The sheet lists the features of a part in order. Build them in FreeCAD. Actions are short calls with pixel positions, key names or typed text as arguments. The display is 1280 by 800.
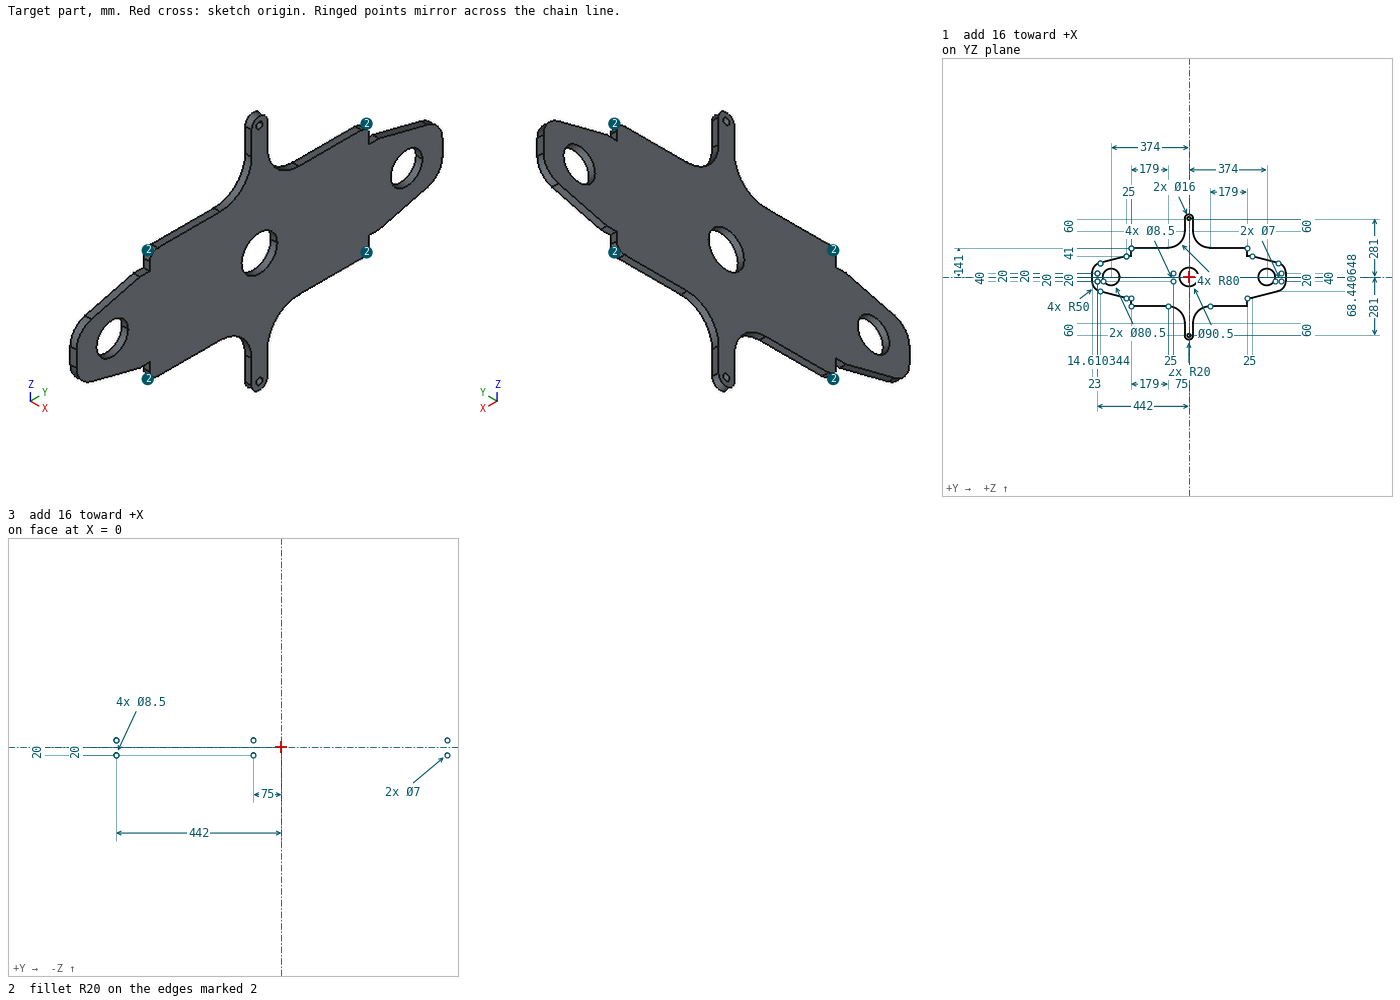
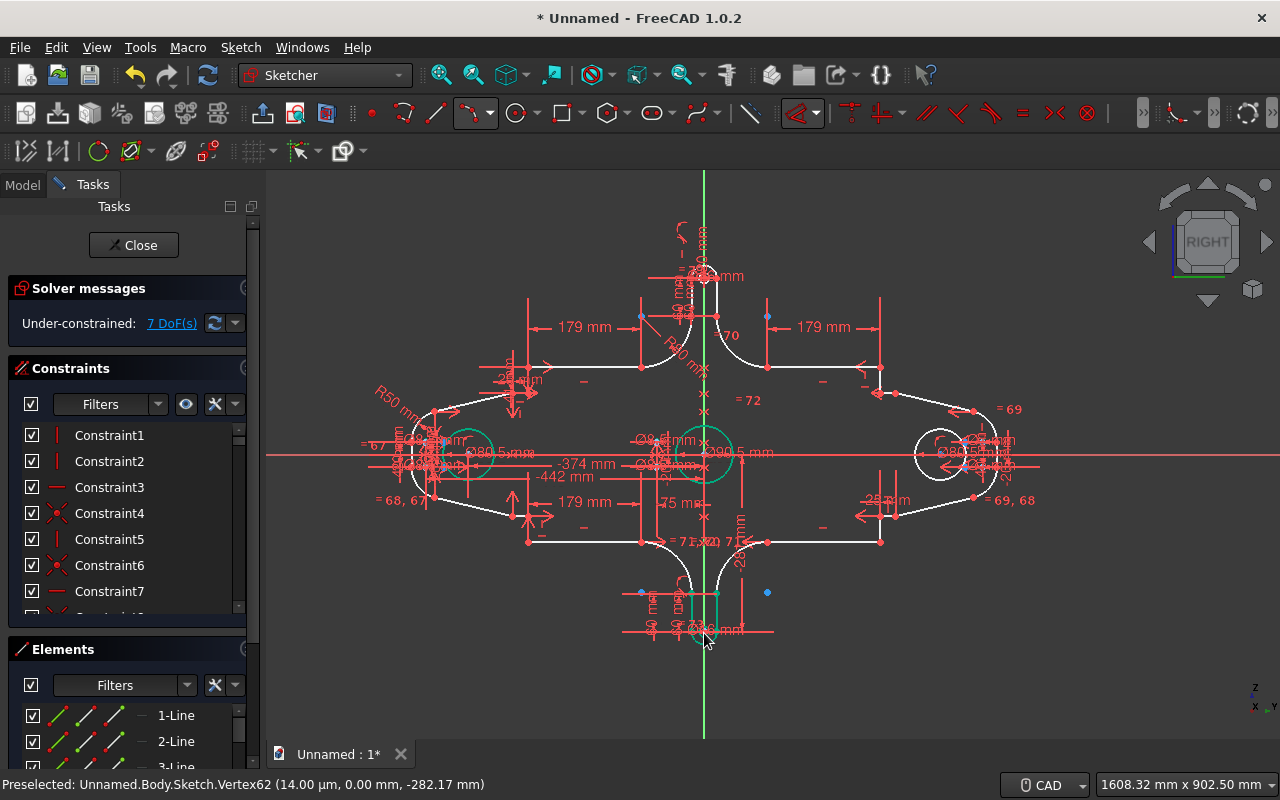
click(704, 278)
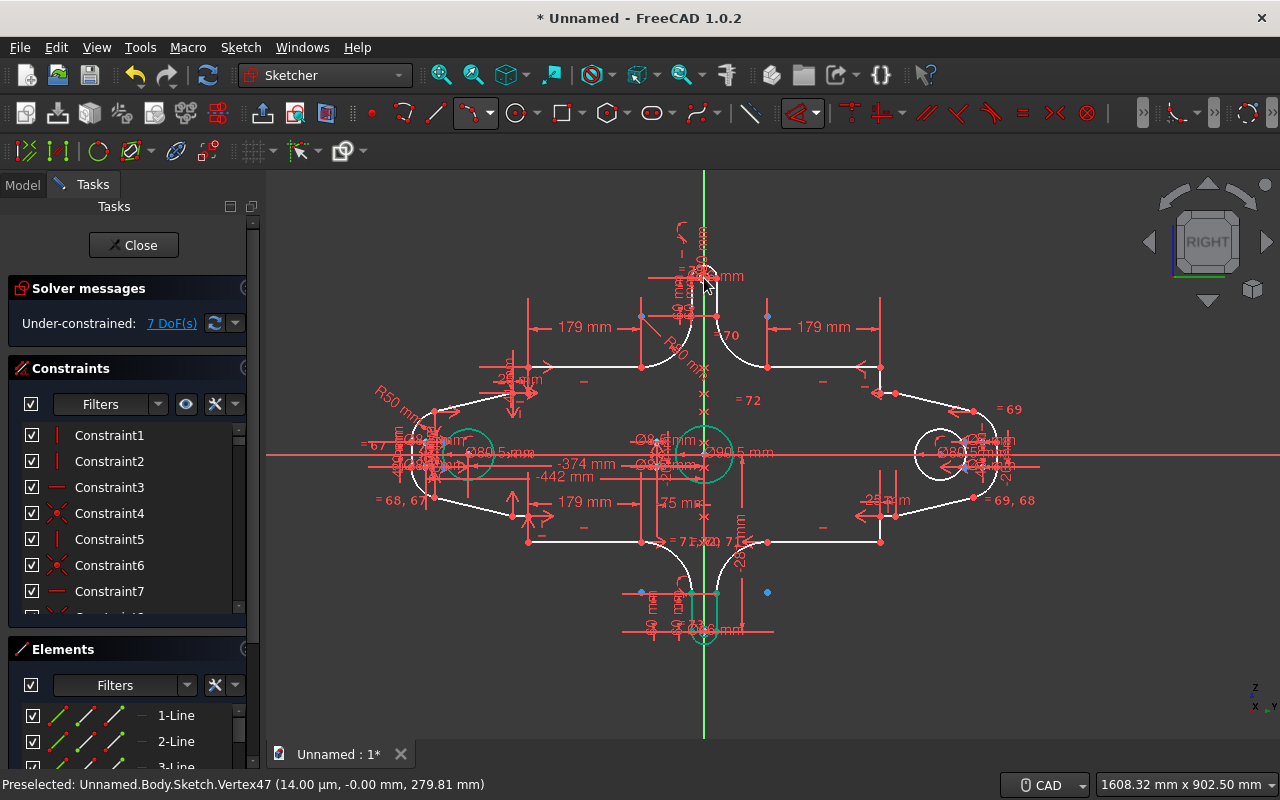
click(818, 114)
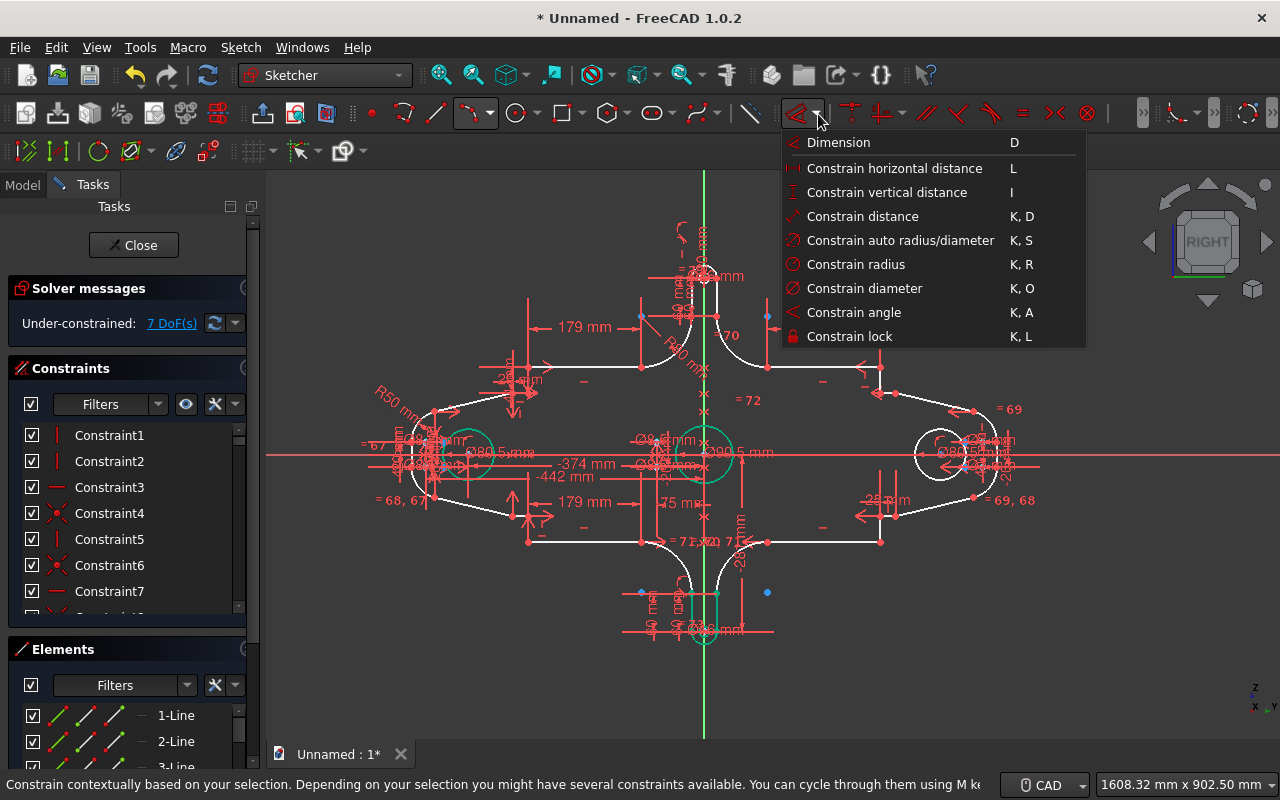
click(934, 192)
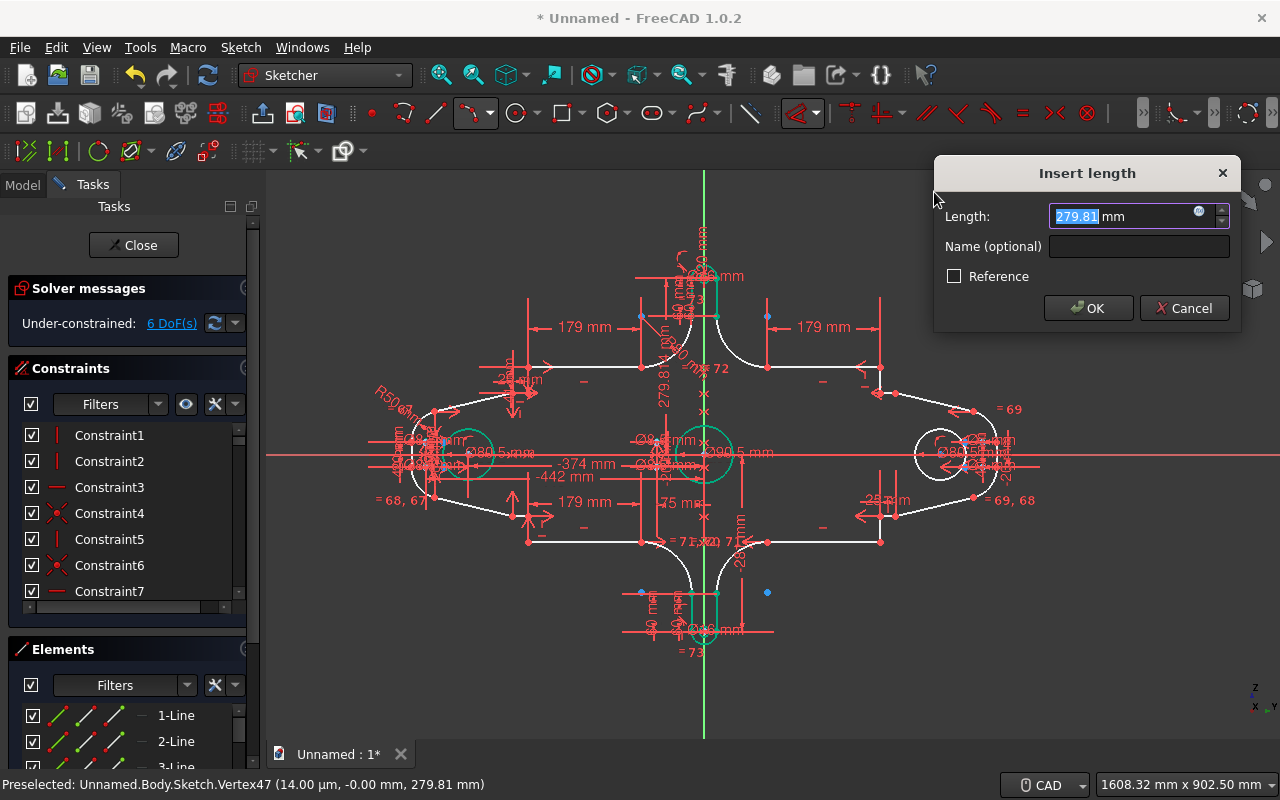
text(281)
key(Return)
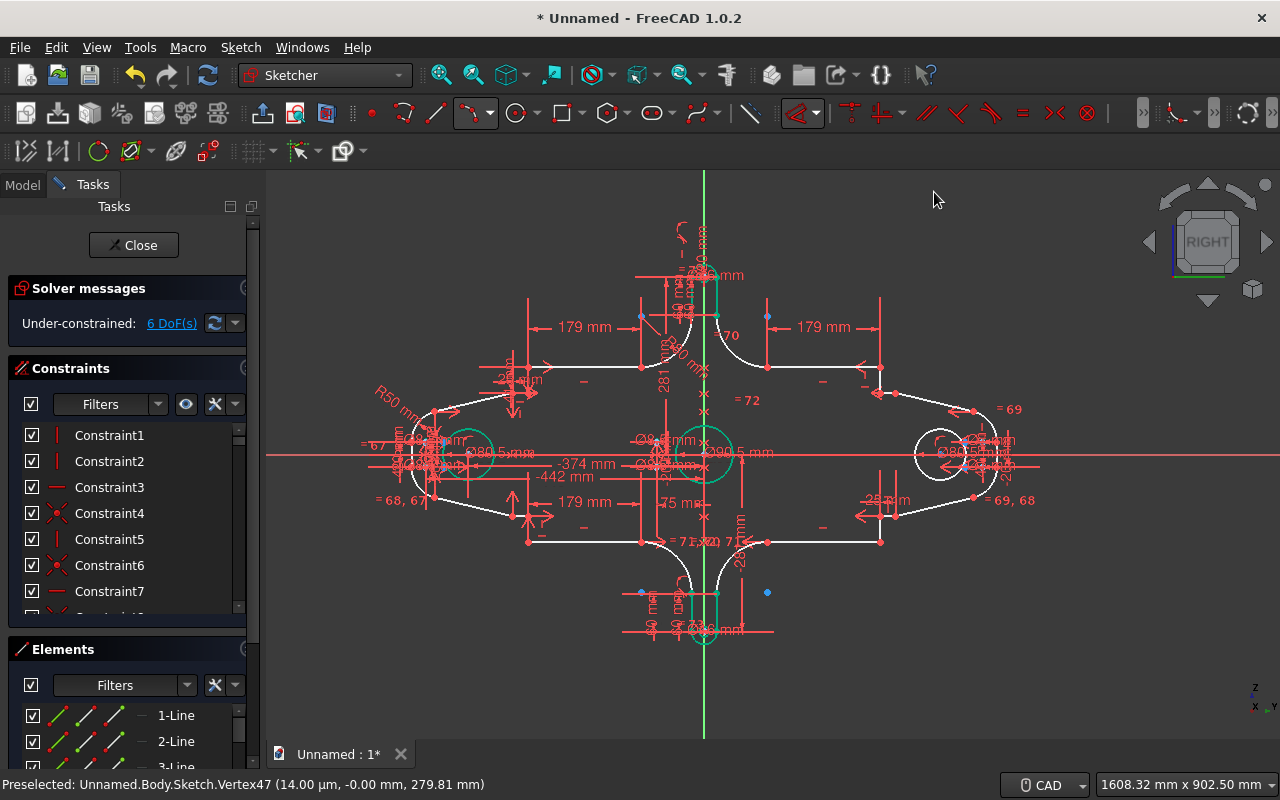
click(940, 455)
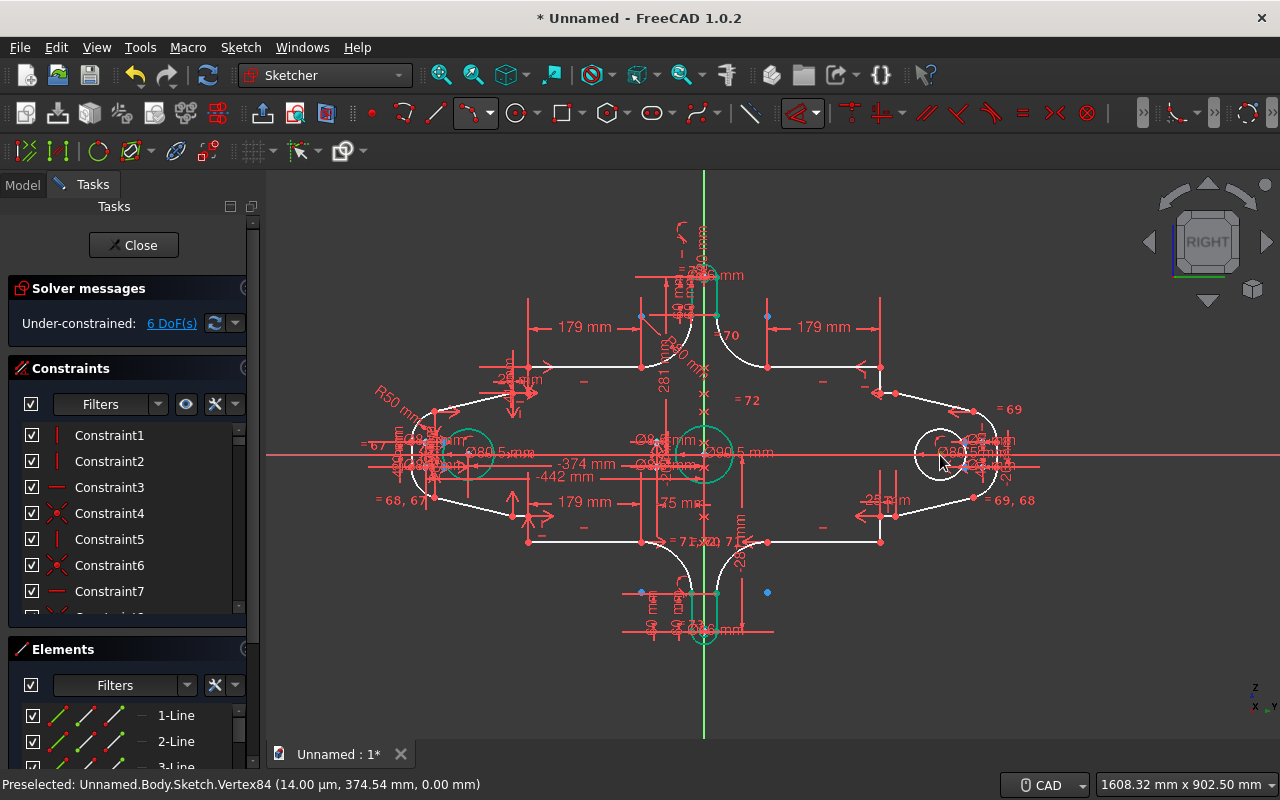
key(l)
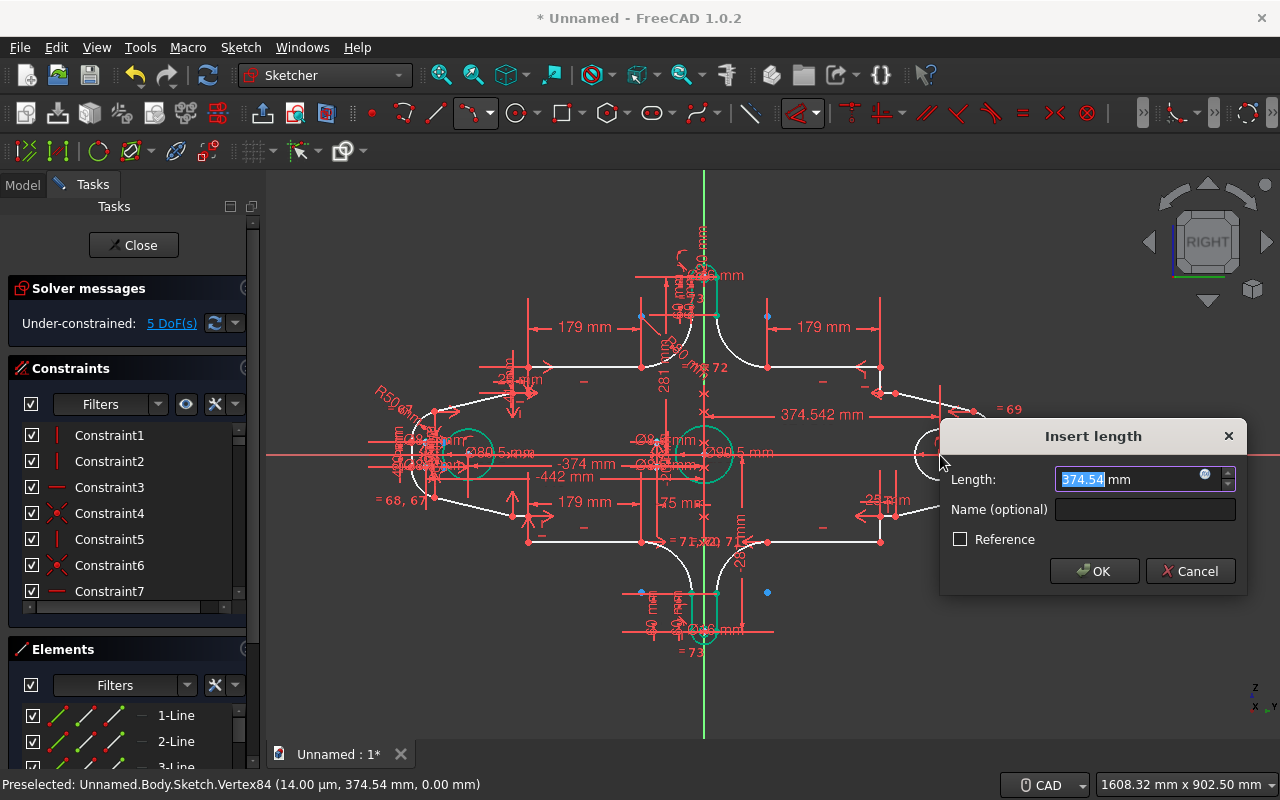
text(374)
key(Return)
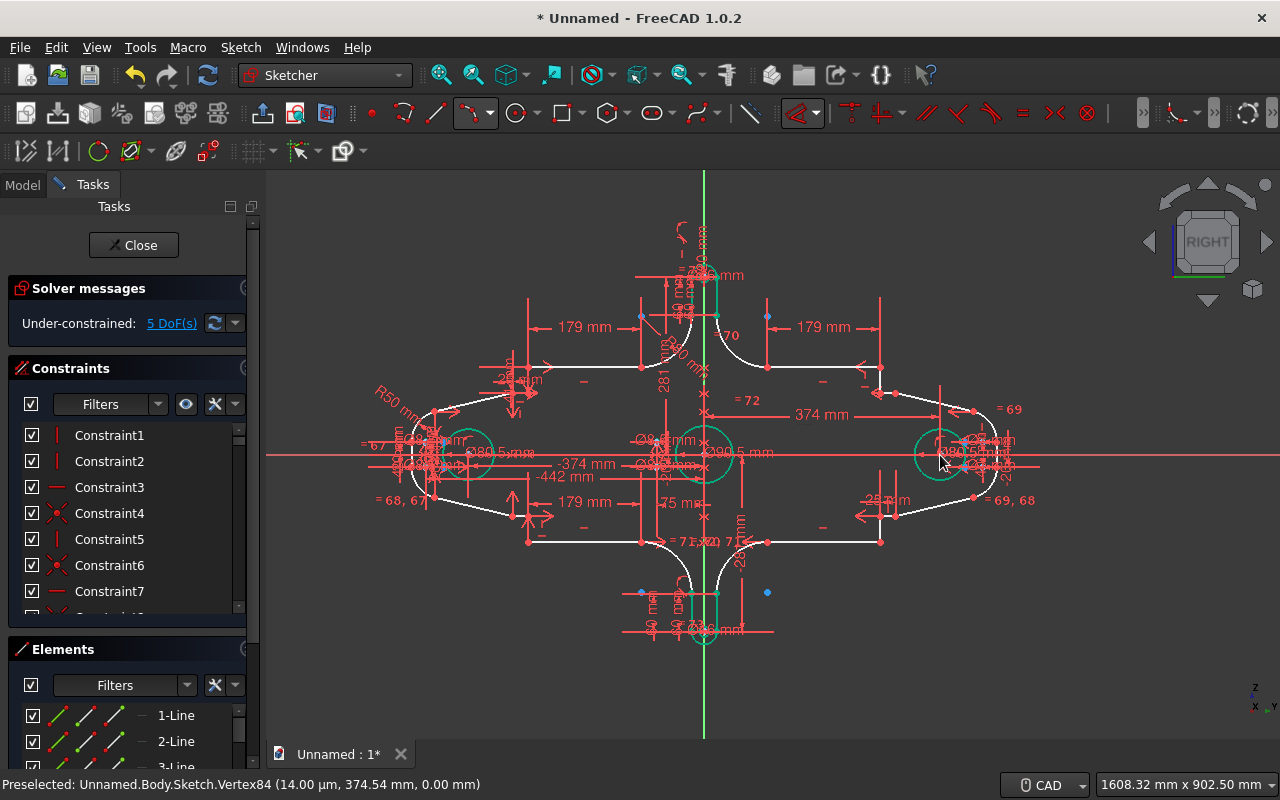
scroll(412, 467, up, 6)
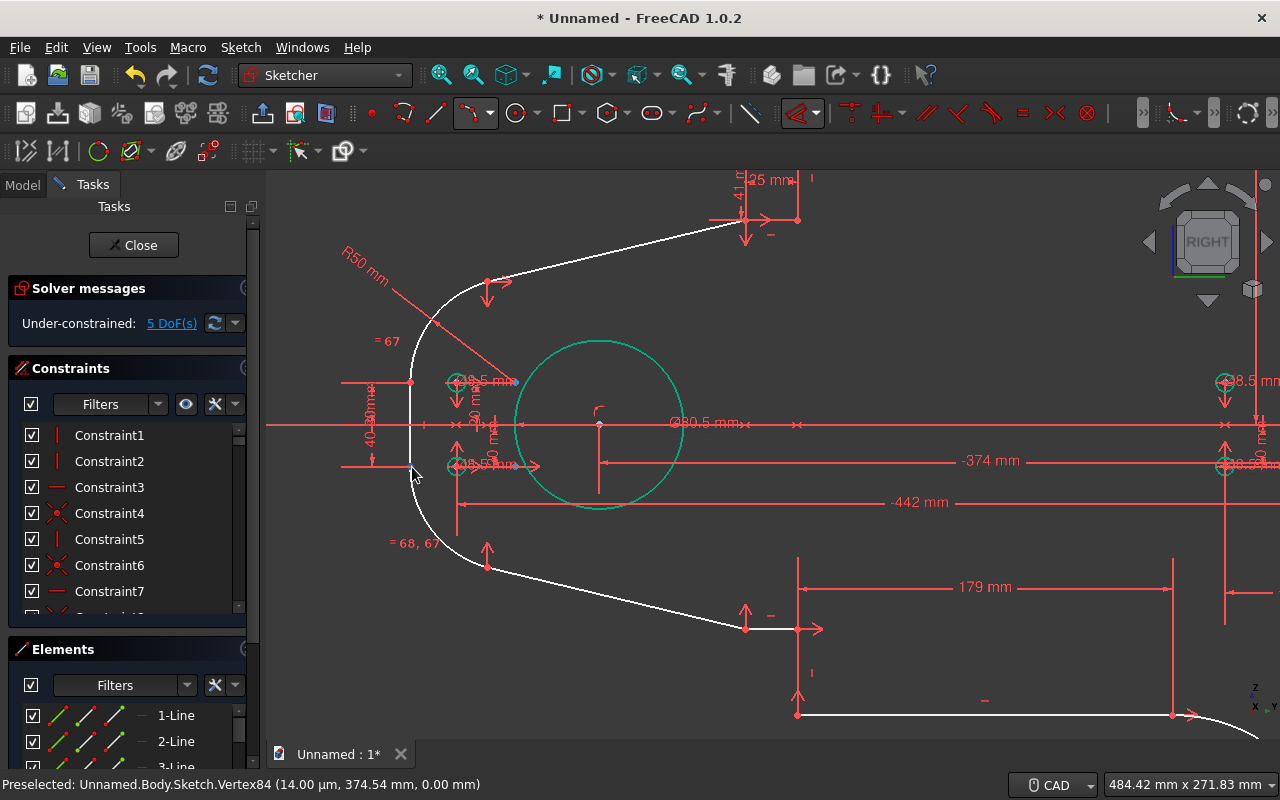
click(410, 467)